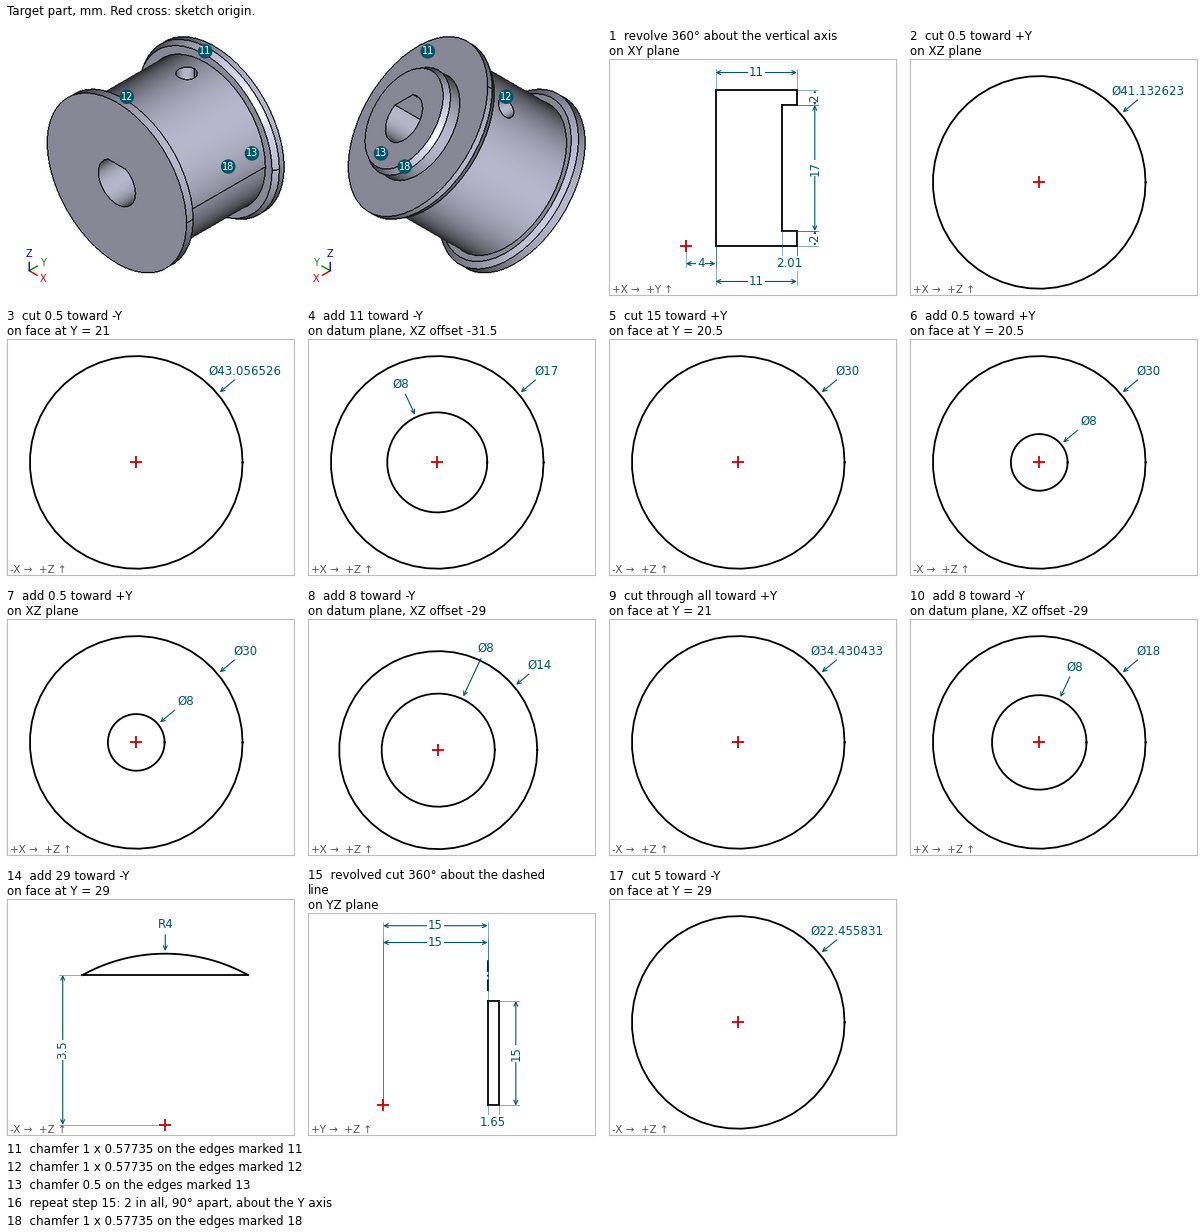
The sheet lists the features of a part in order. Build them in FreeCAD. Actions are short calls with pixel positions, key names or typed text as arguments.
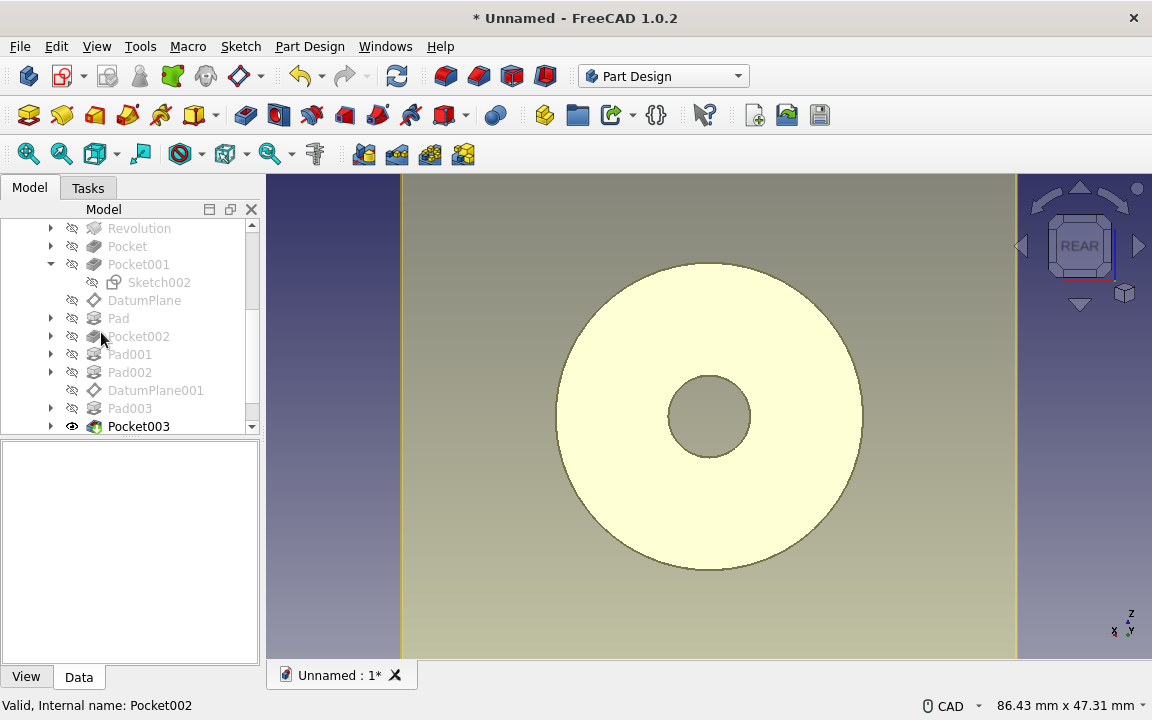
scroll(141, 332, up, 15)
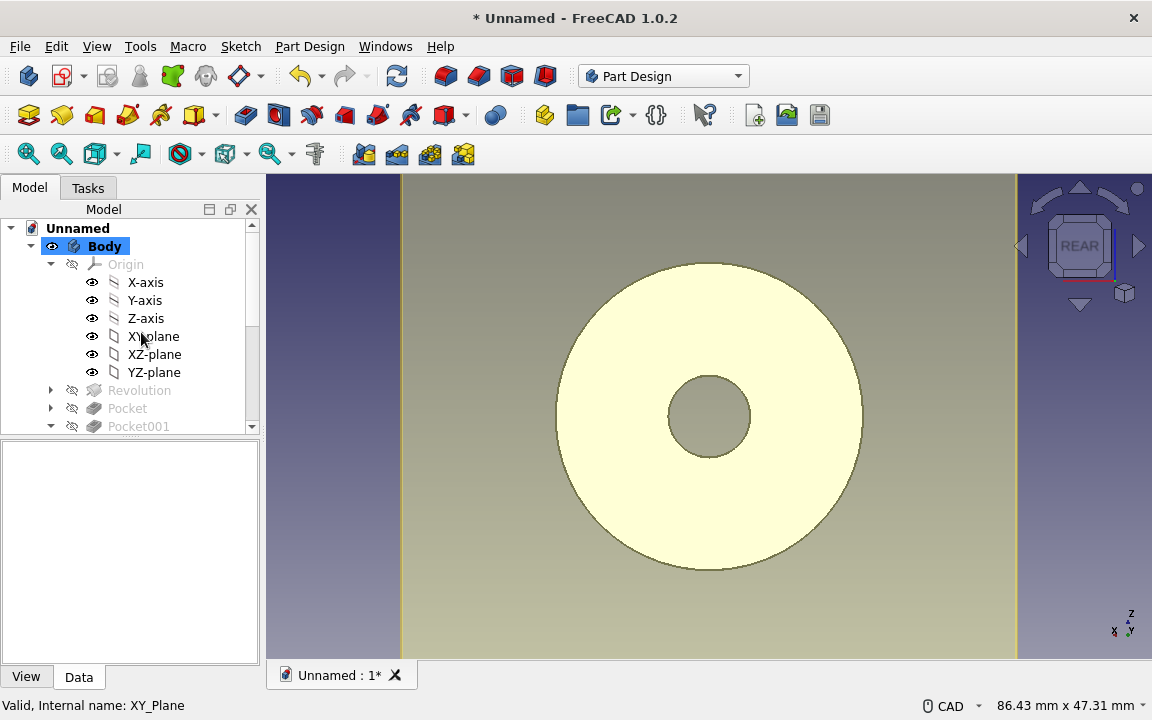
scroll(101, 332, down, 6)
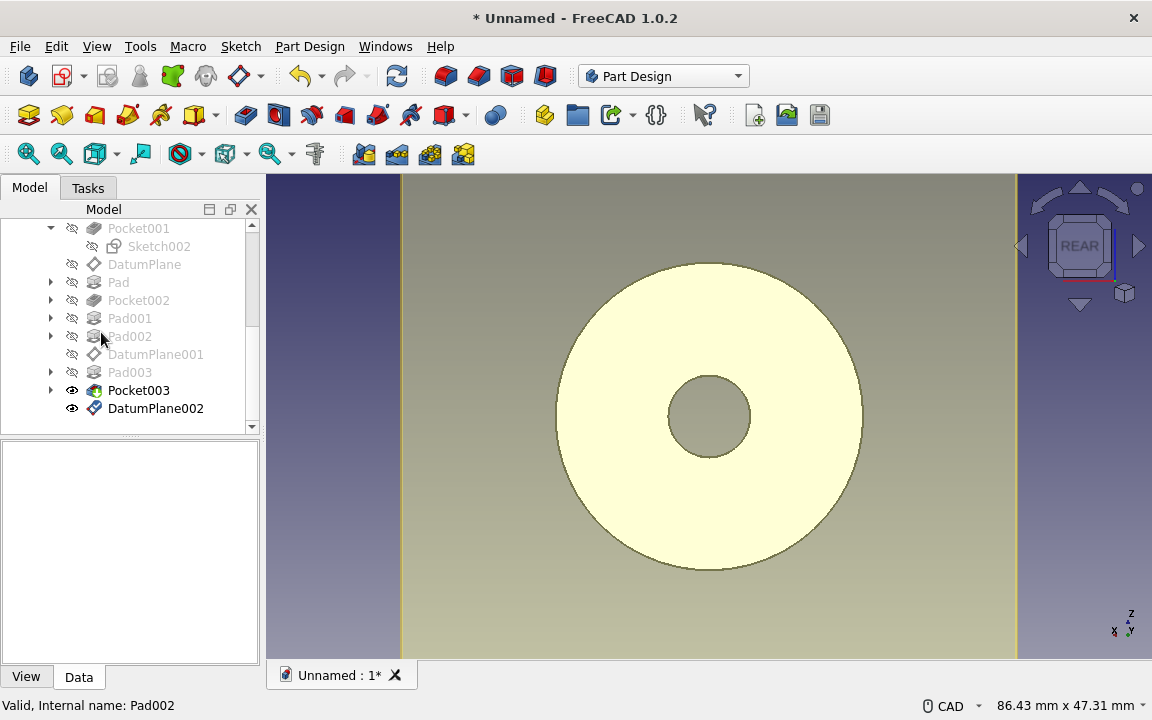
click(117, 408)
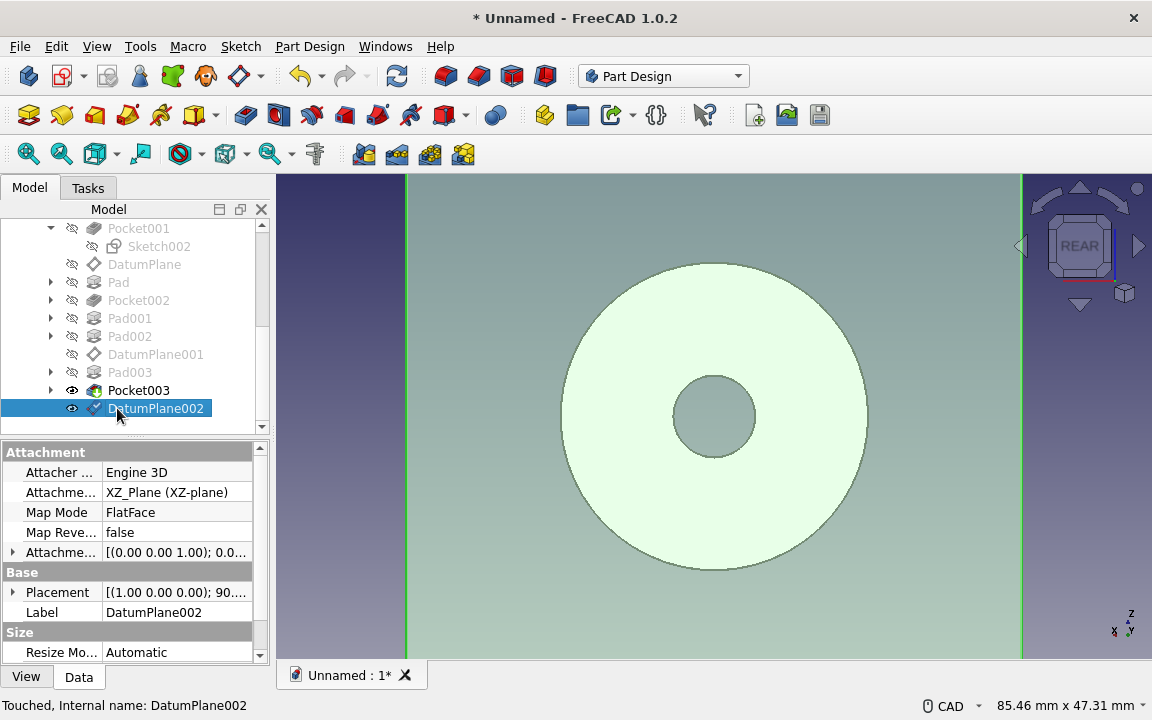
click(62, 76)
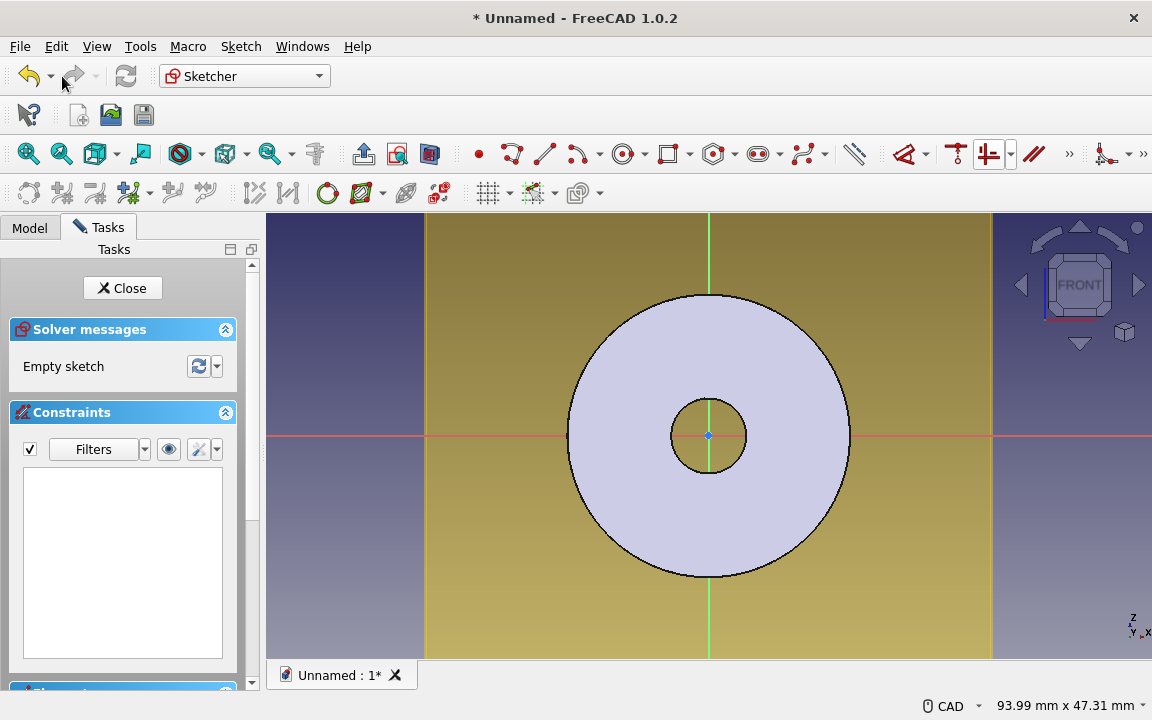
click(430, 154)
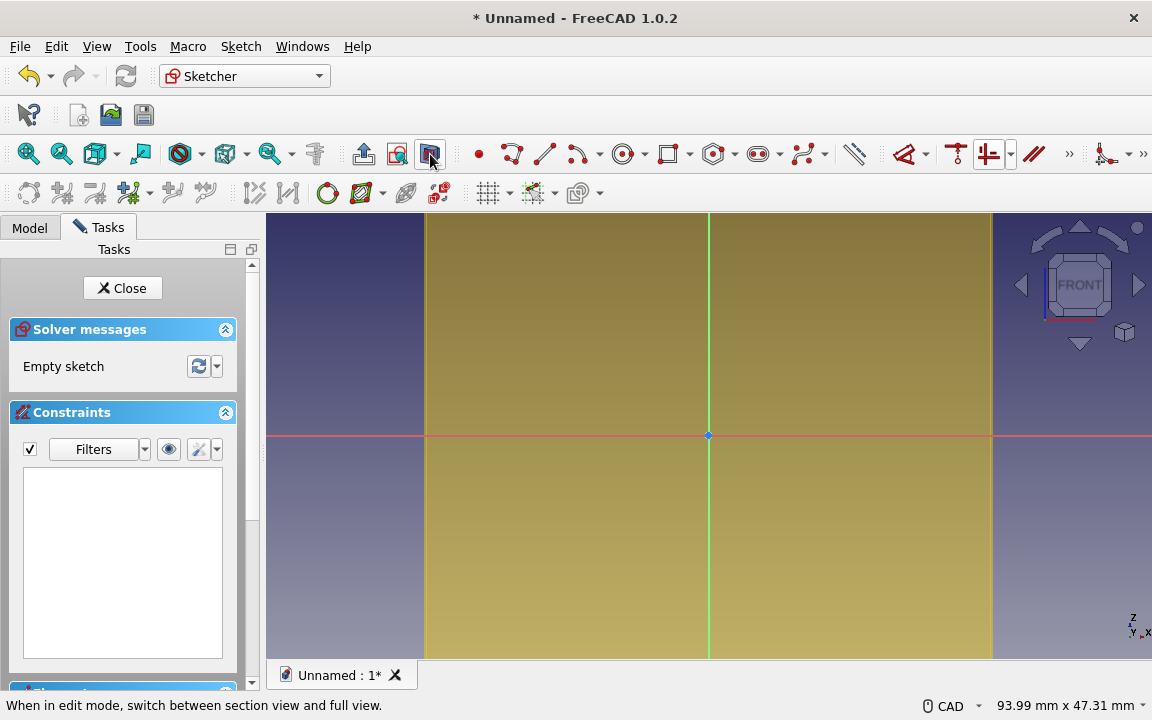
scroll(847, 436, up, 2)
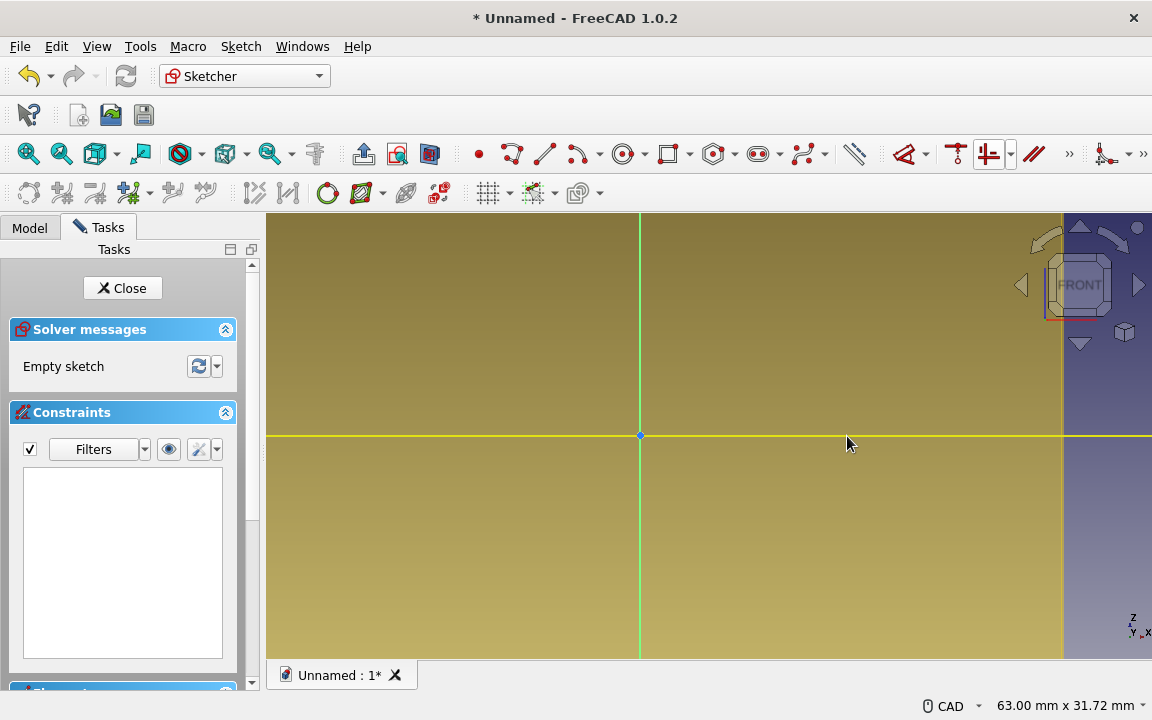
click(622, 154)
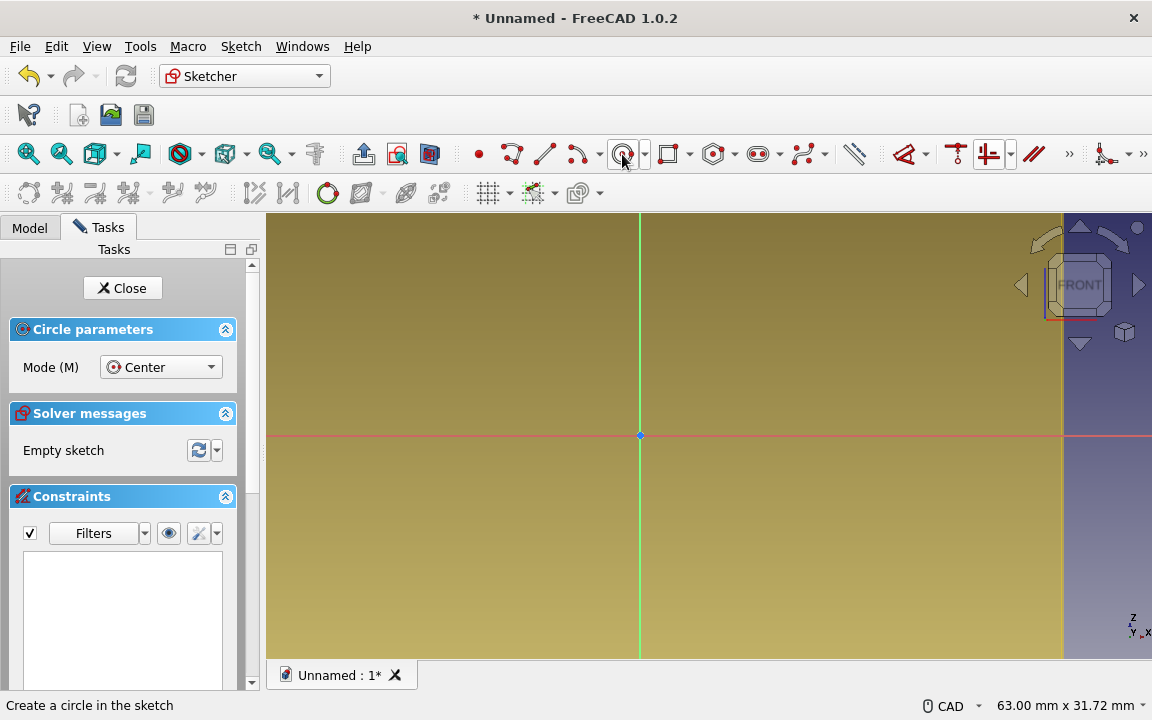
click(640, 436)
move(730, 346)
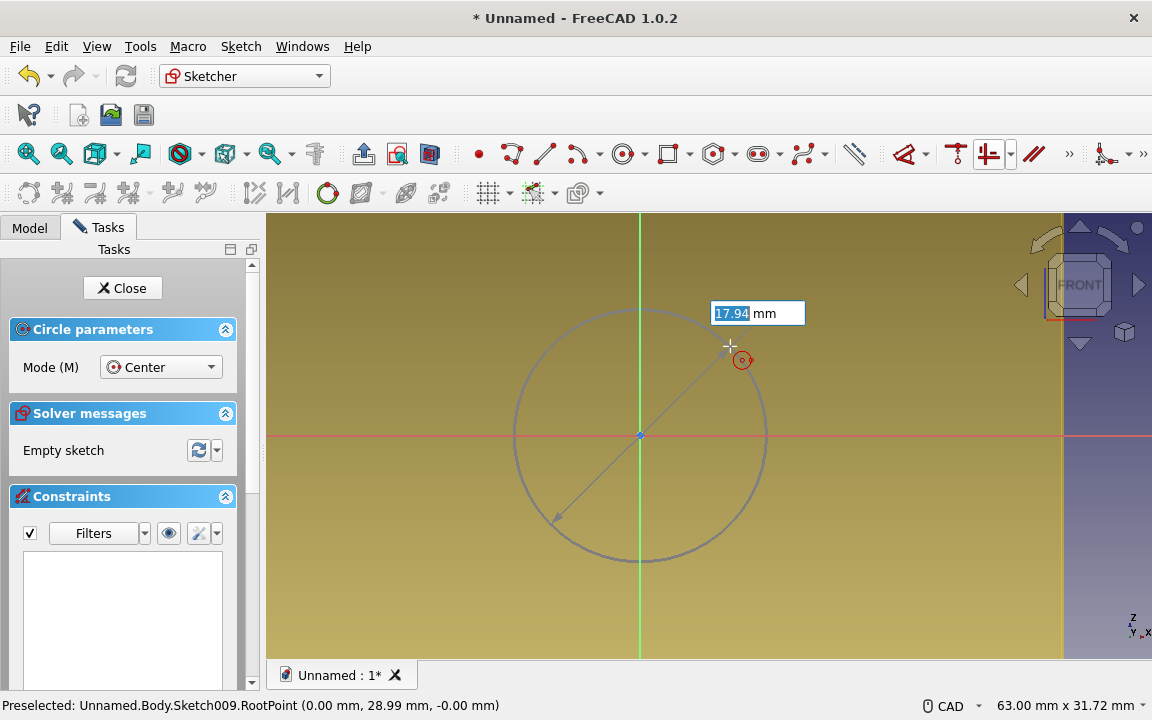
text(18)
key(Return)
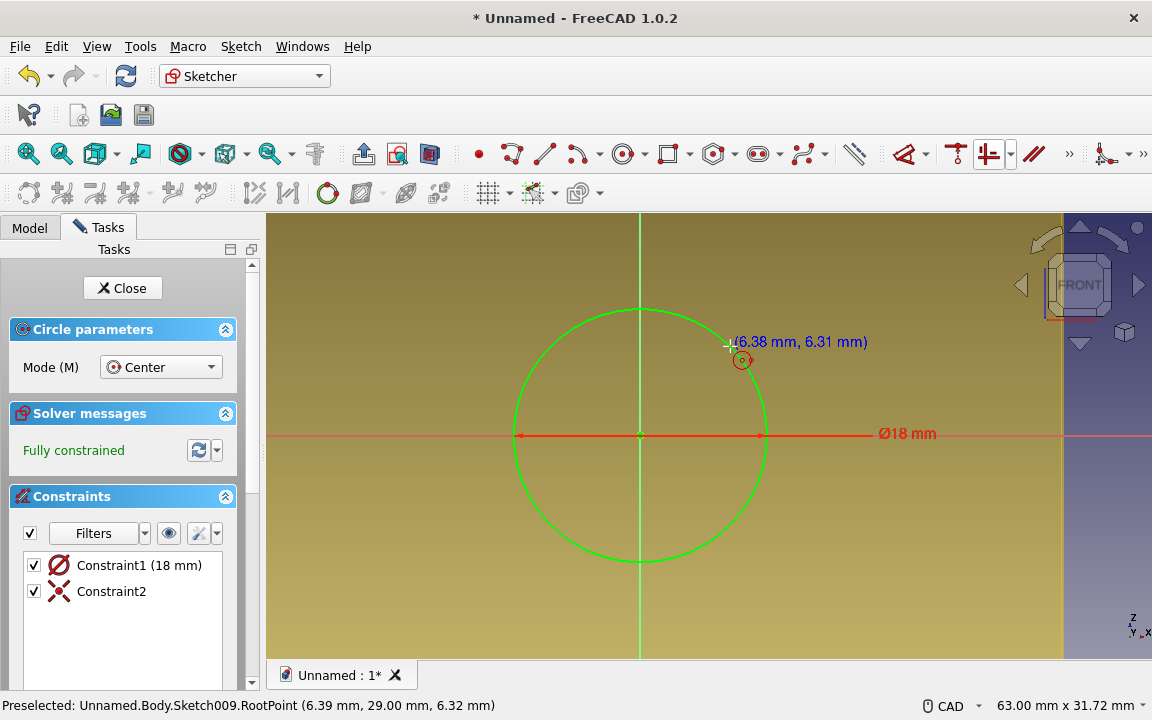
click(640, 436)
move(680, 396)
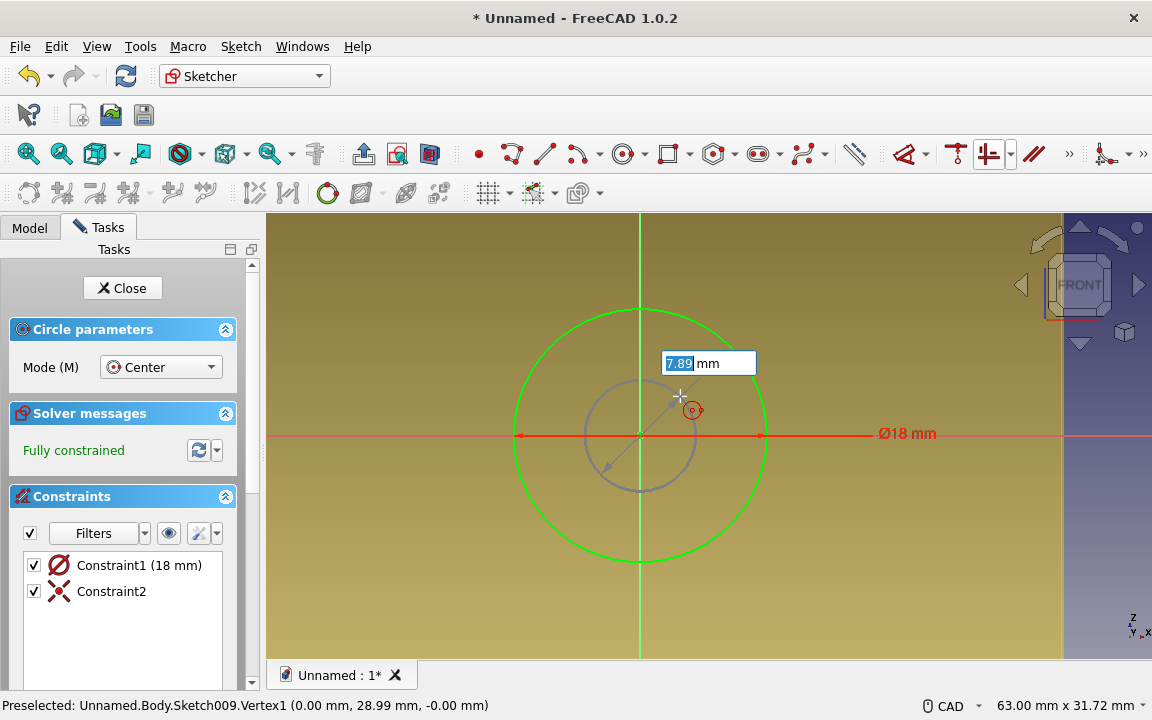
text(8)
key(Return)
key(Escape)